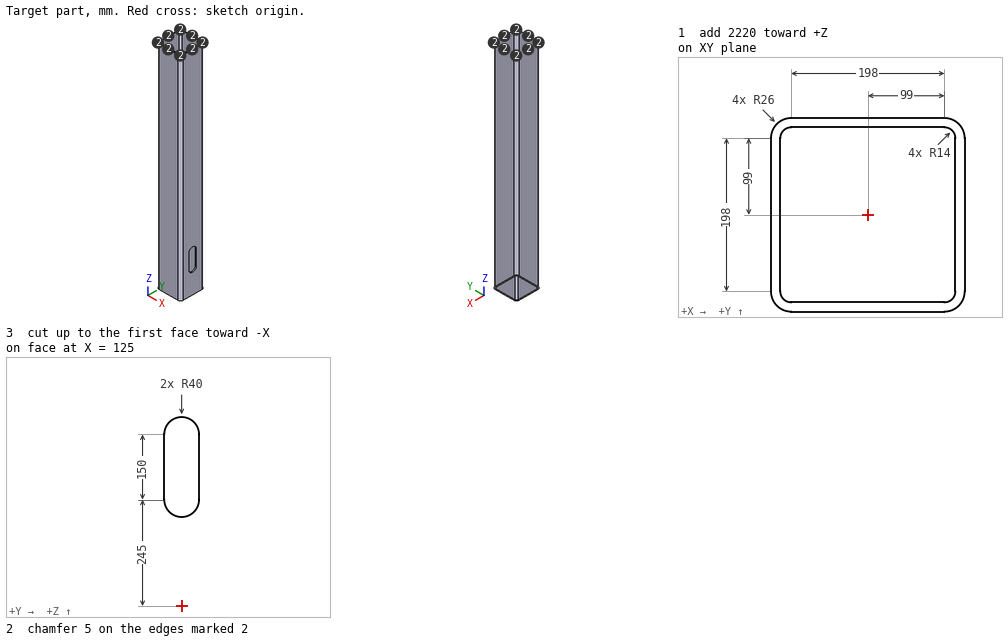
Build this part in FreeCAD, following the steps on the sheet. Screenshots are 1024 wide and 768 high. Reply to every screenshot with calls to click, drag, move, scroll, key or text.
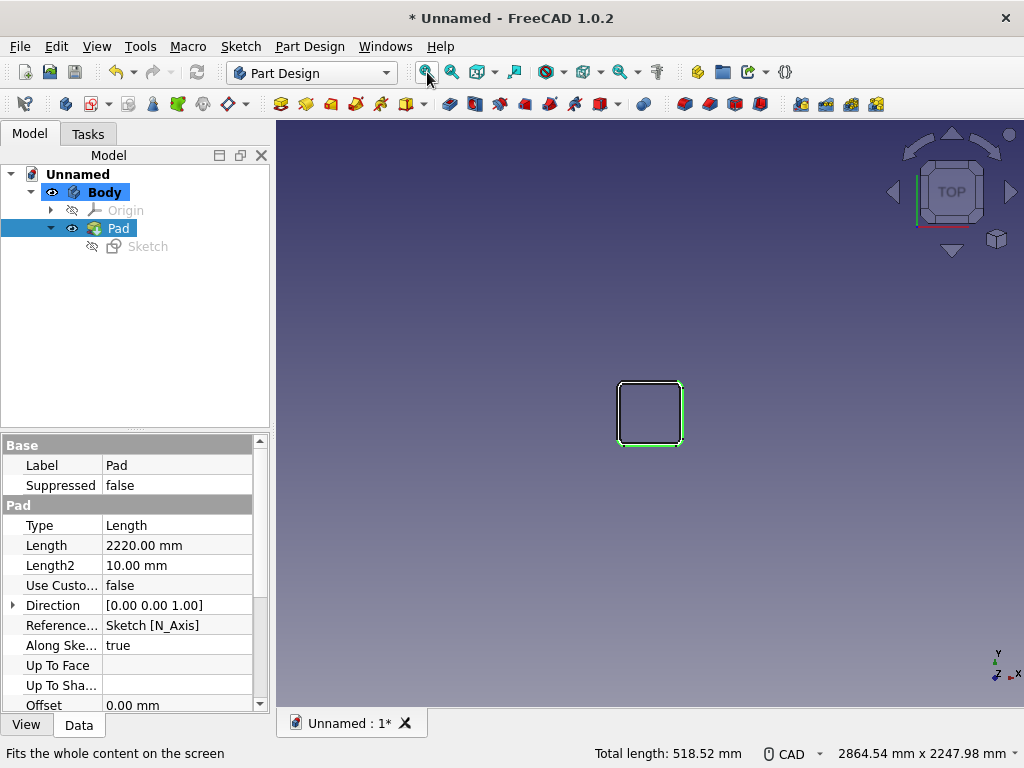
click(650, 380, ctrl)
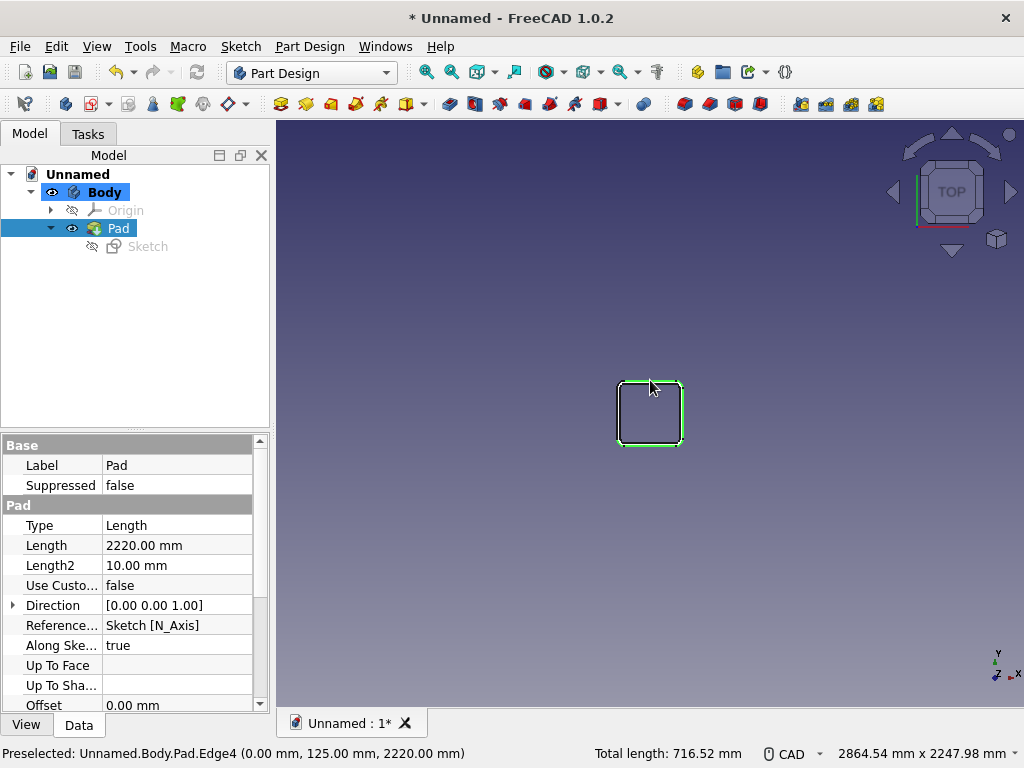
click(617, 412, ctrl)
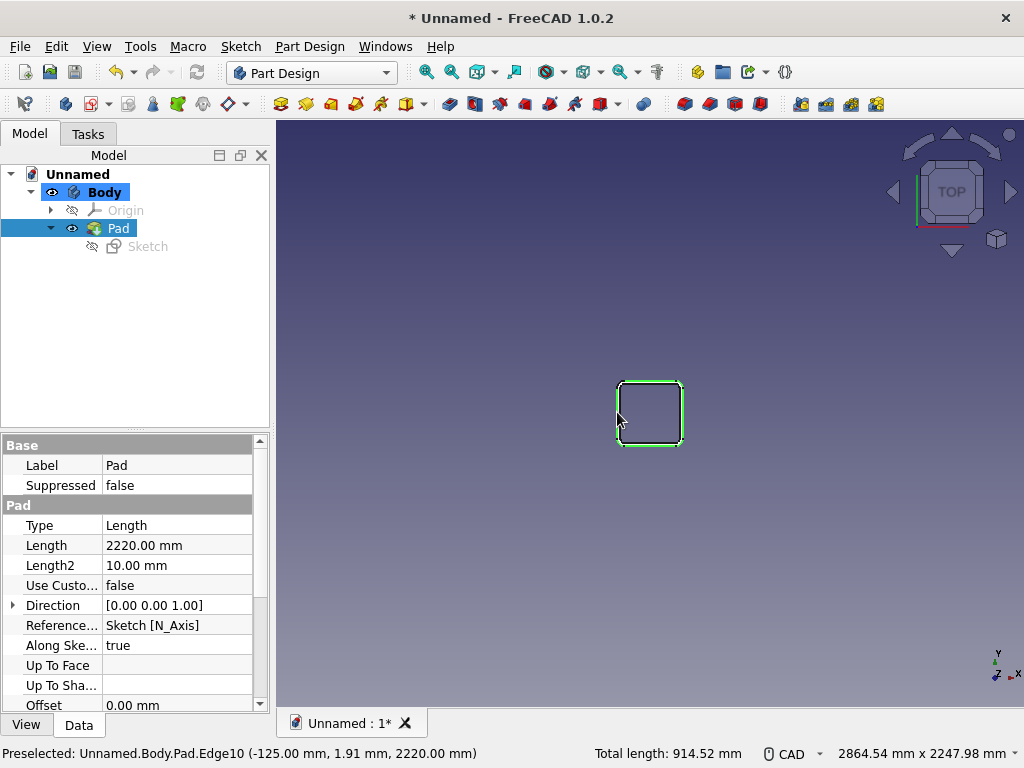
scroll(619, 382, up, 7)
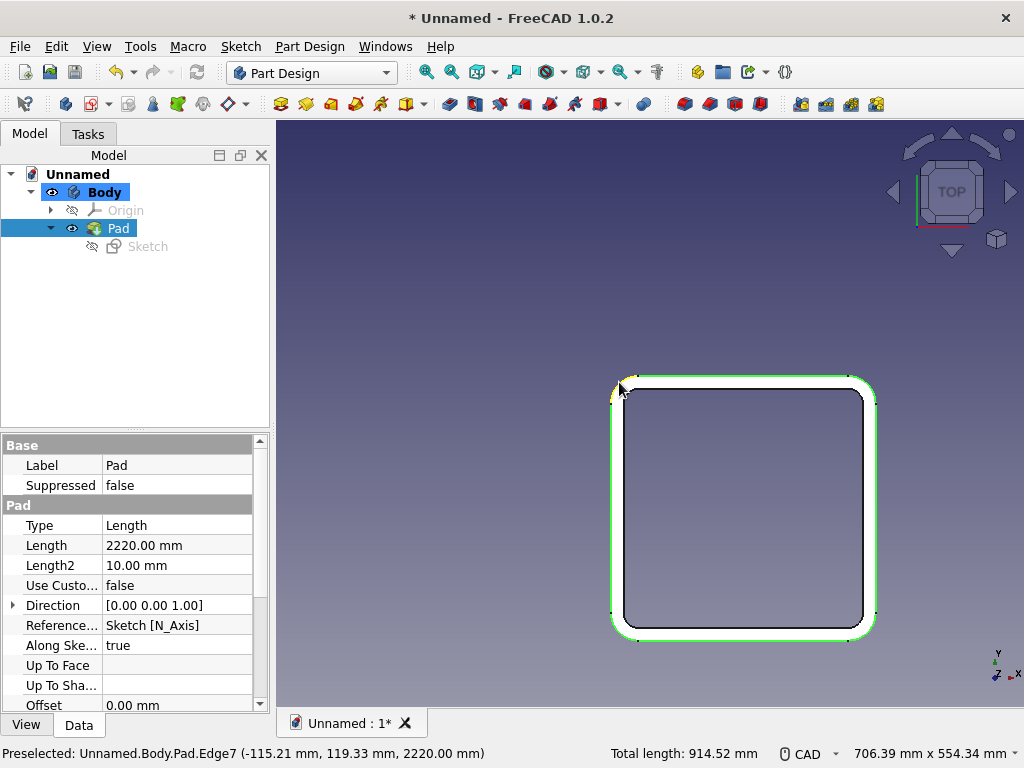
click(619, 383, ctrl)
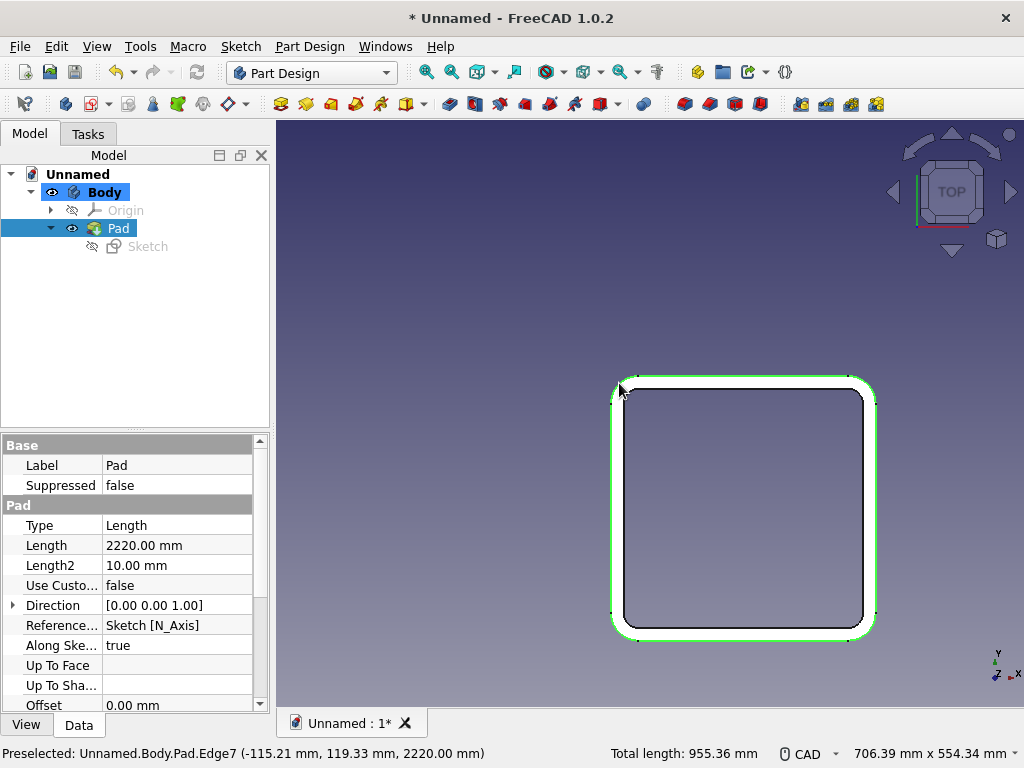
click(710, 104)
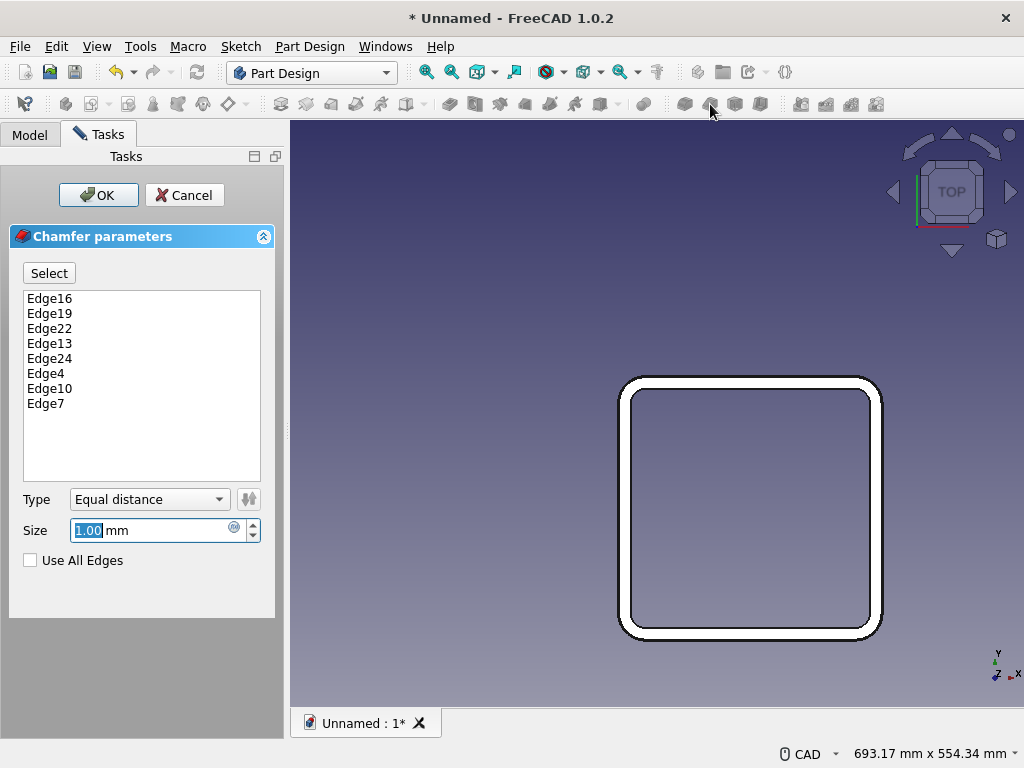
text(5)
key(Tab)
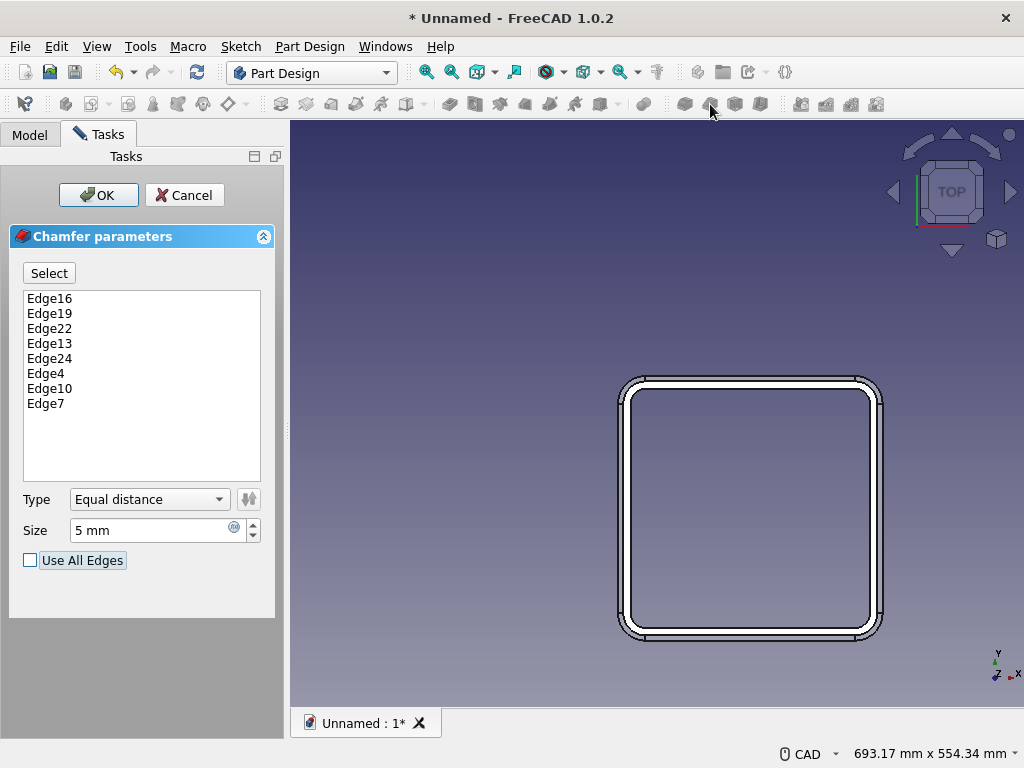
click(99, 195)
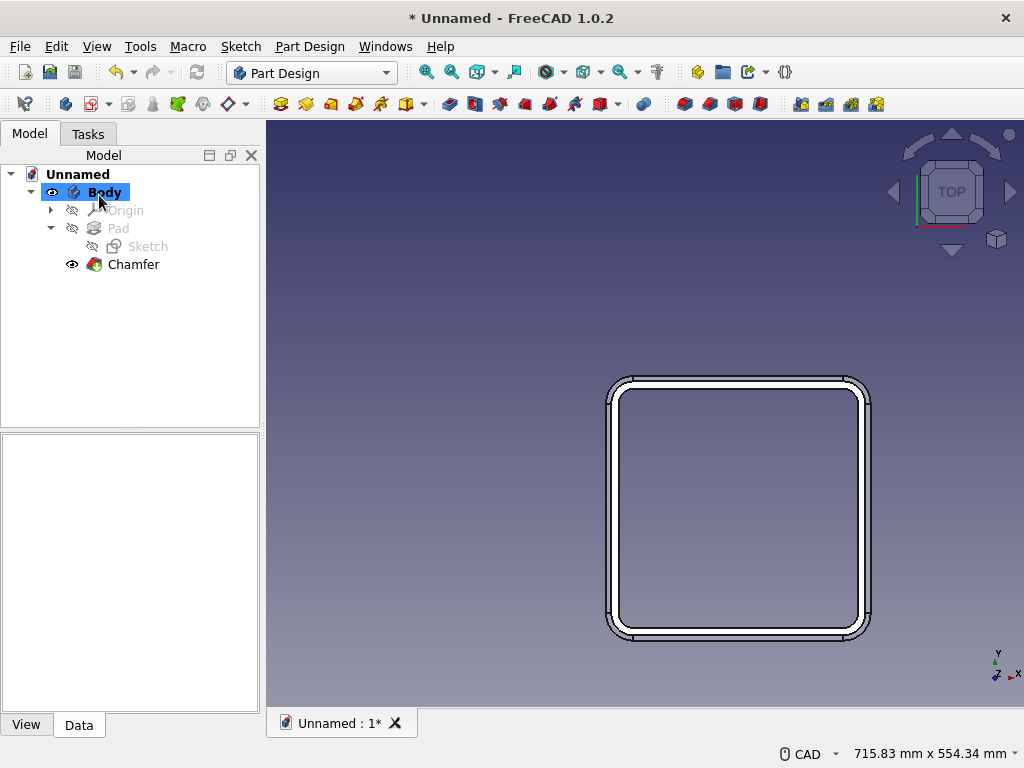
key(0)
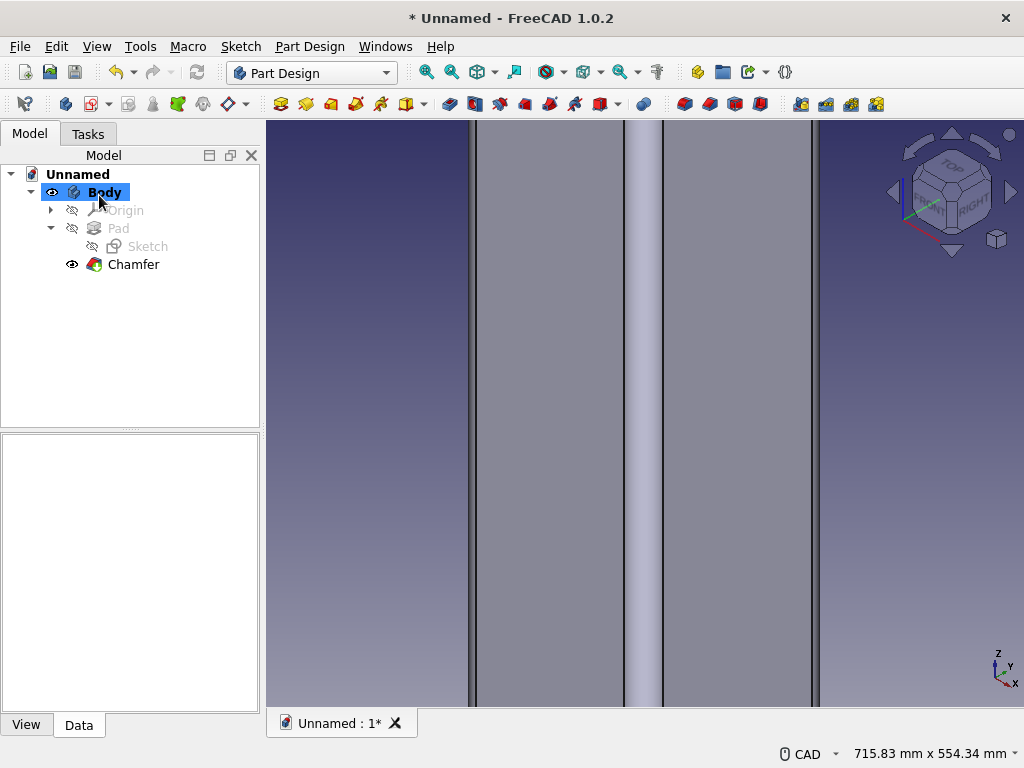
click(427, 72)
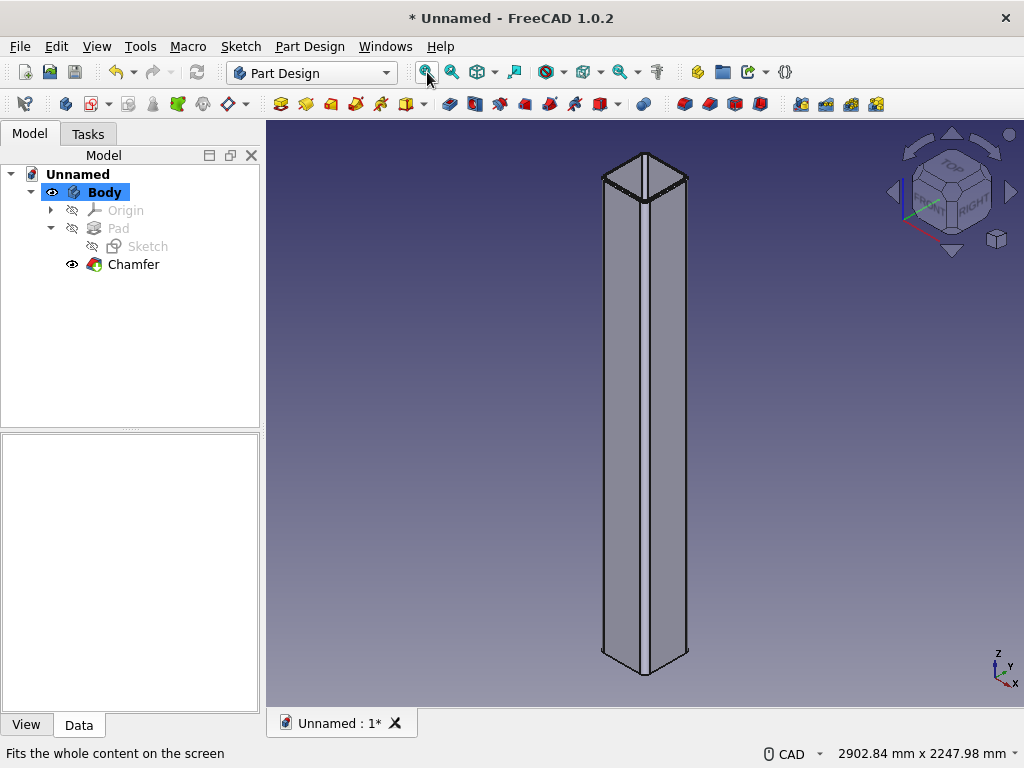
click(668, 224)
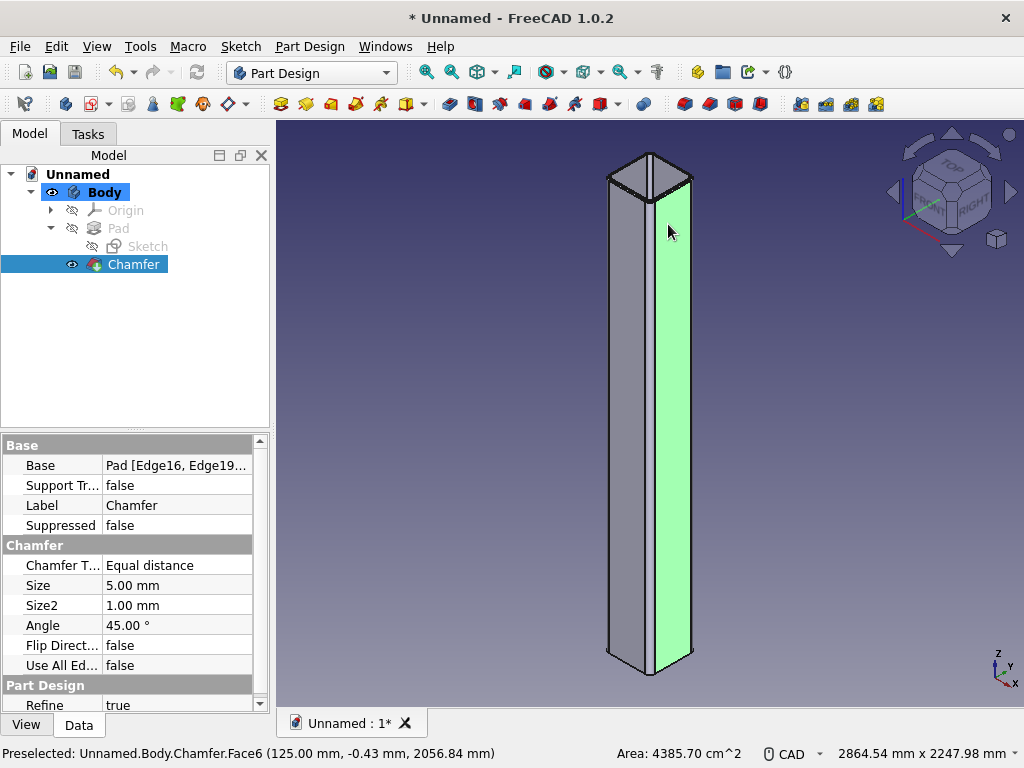
click(90, 104)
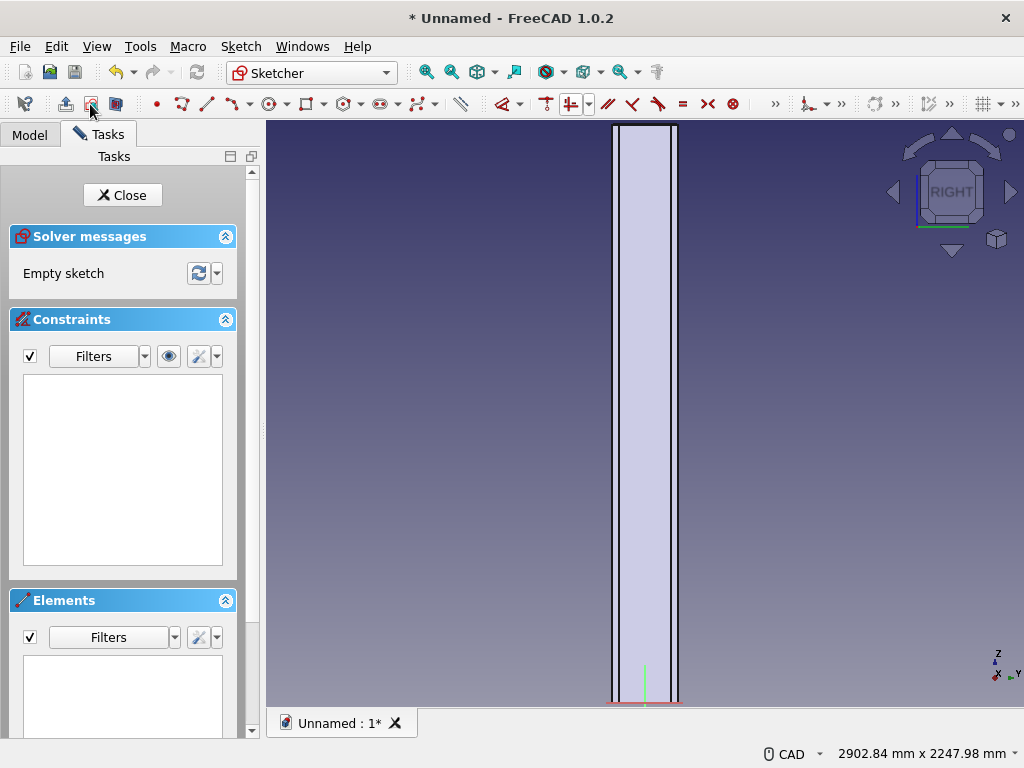
scroll(576, 414, down, 5)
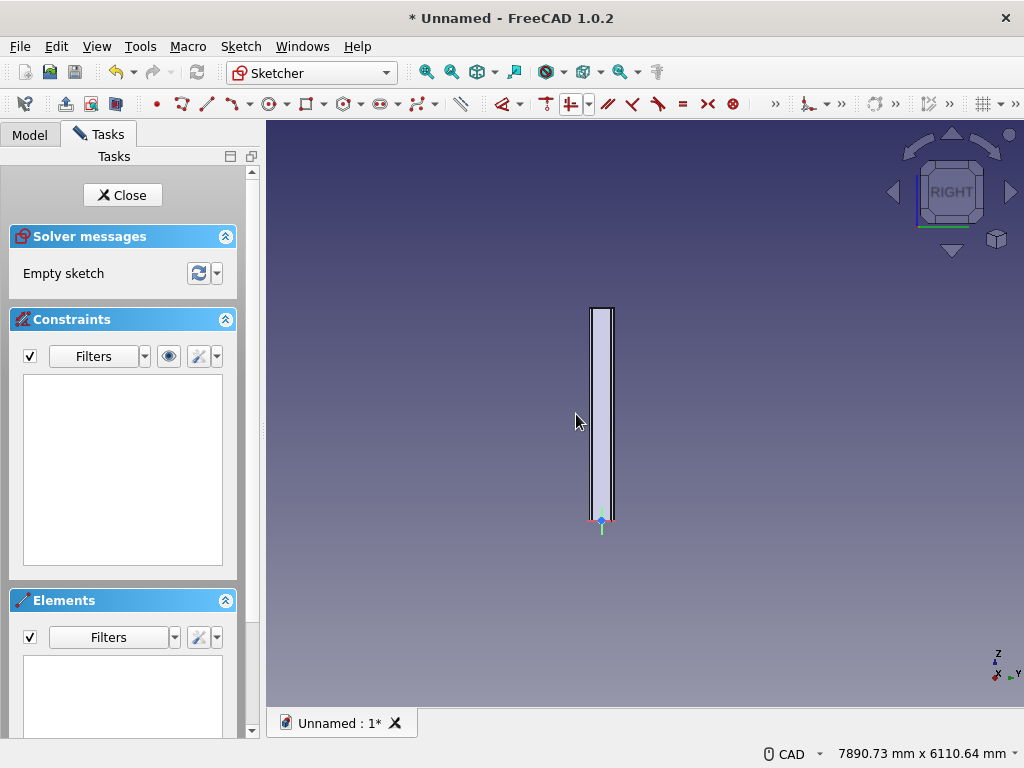
scroll(605, 511, up, 11)